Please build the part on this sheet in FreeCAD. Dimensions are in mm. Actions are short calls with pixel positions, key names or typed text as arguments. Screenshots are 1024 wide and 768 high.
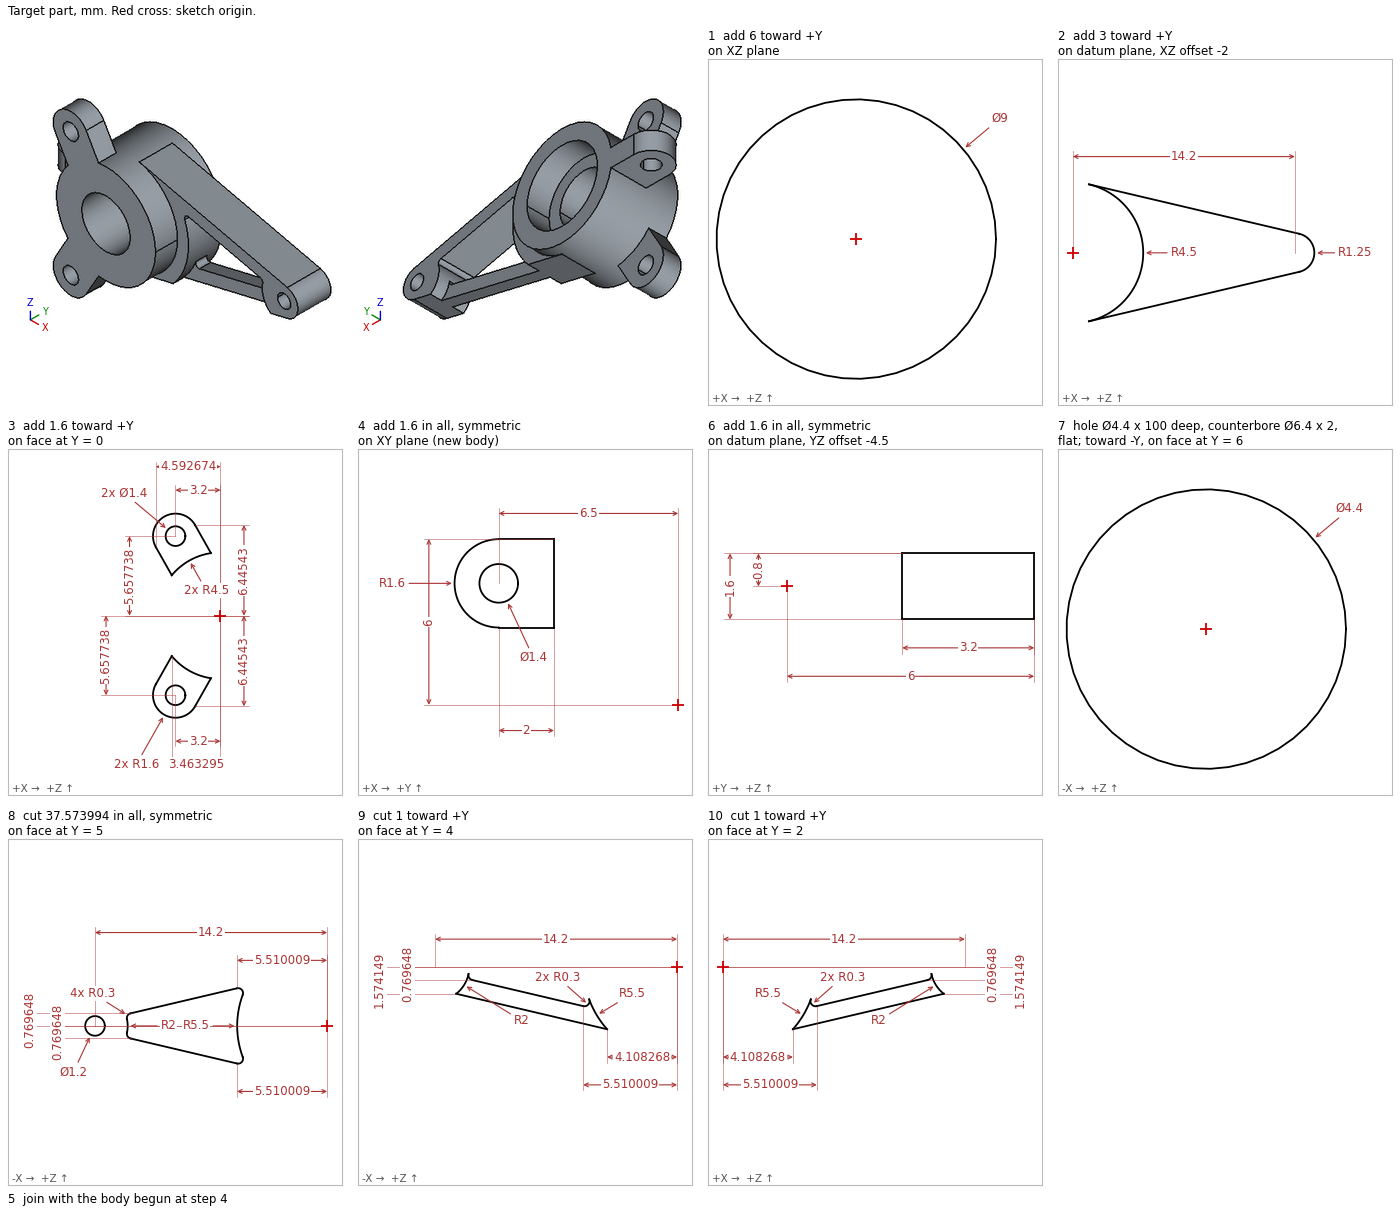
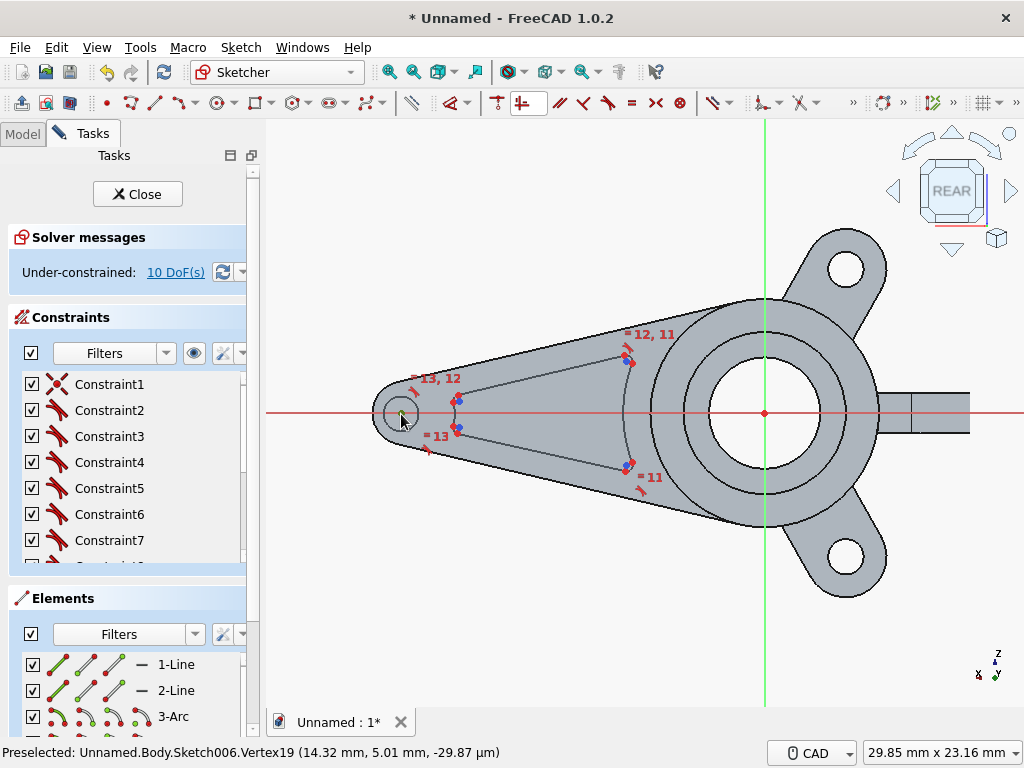
click(334, 413)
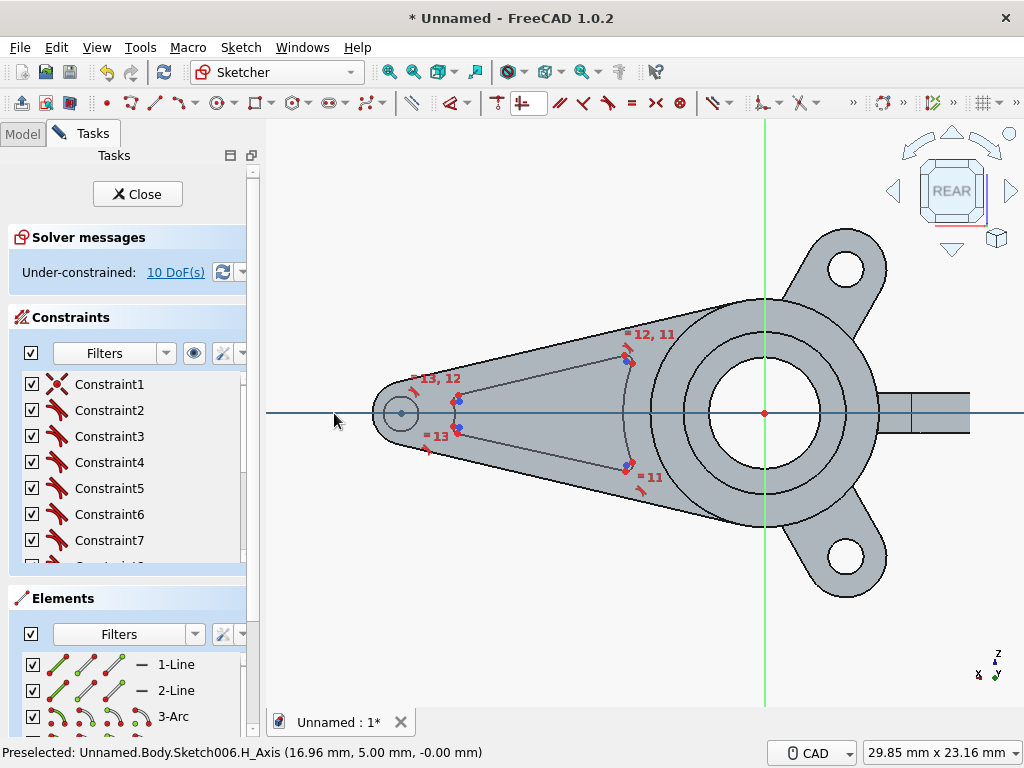
key(c)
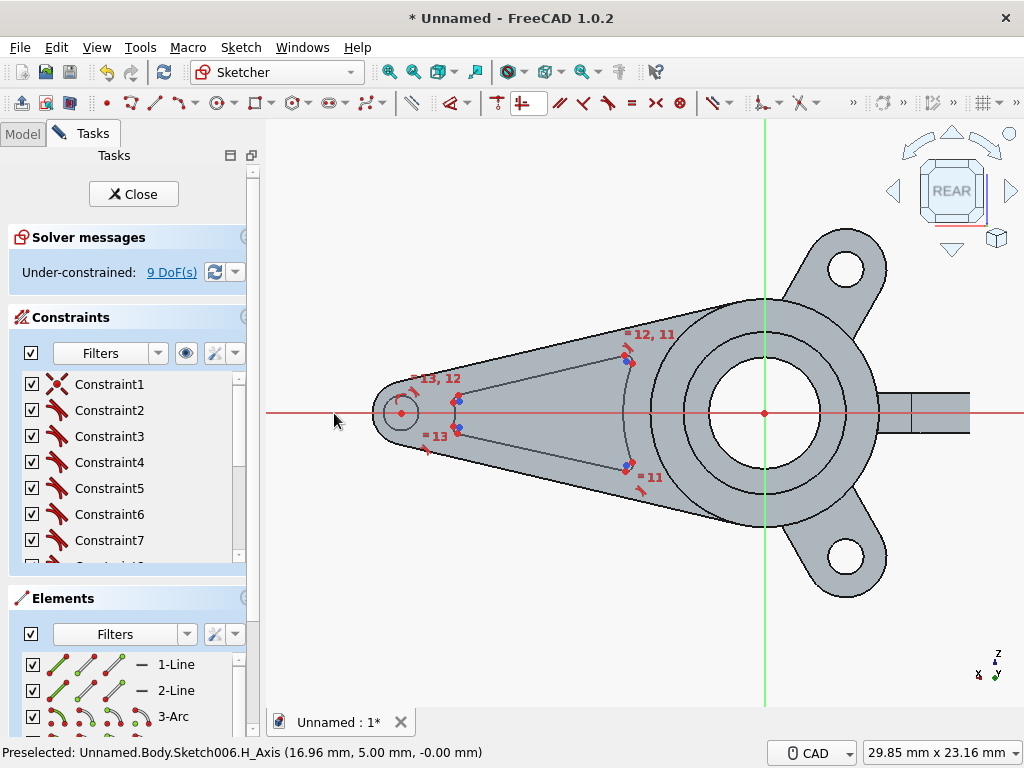
click(450, 104)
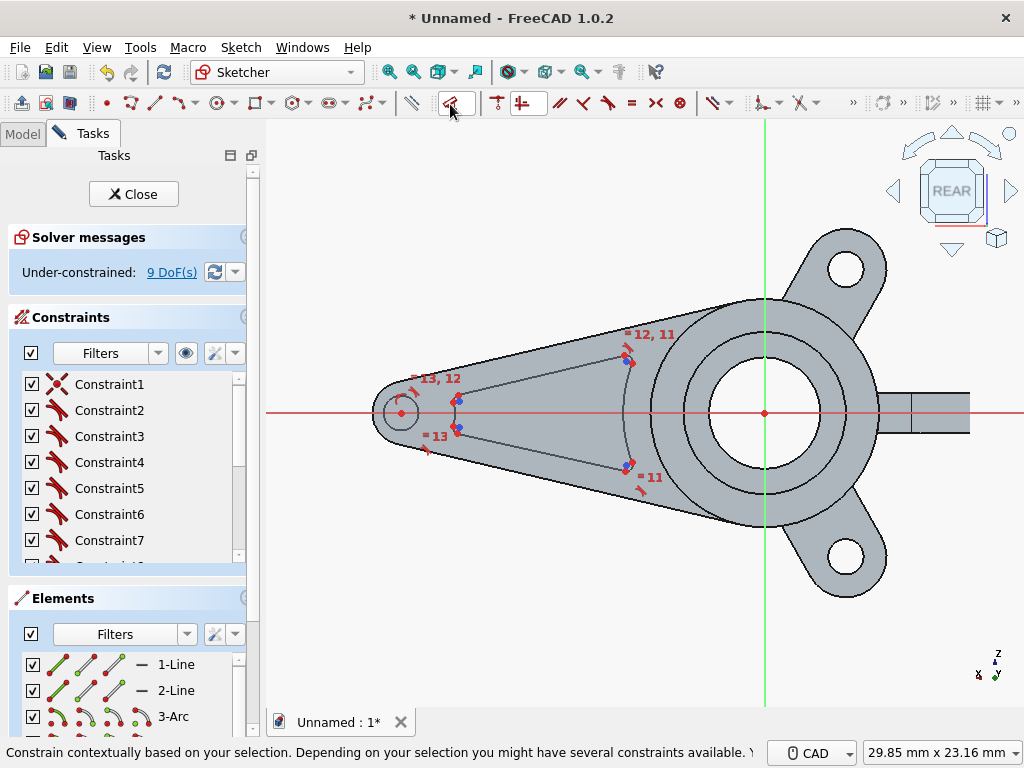
scroll(631, 469, up, 9)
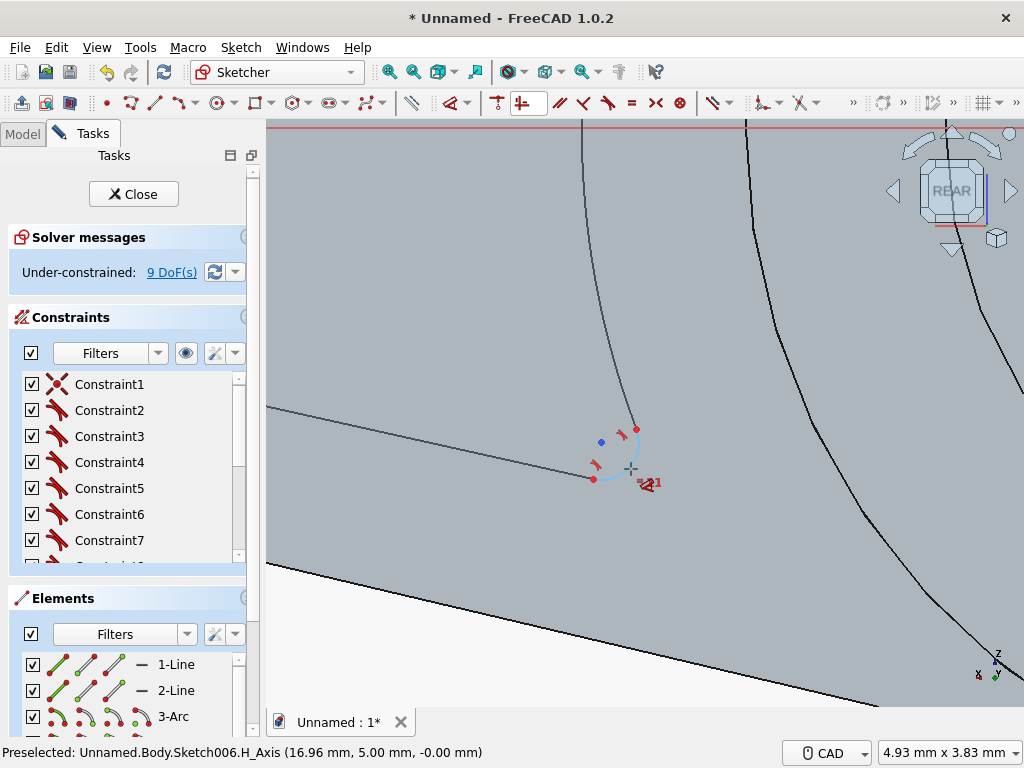
click(630, 467)
click(654, 488)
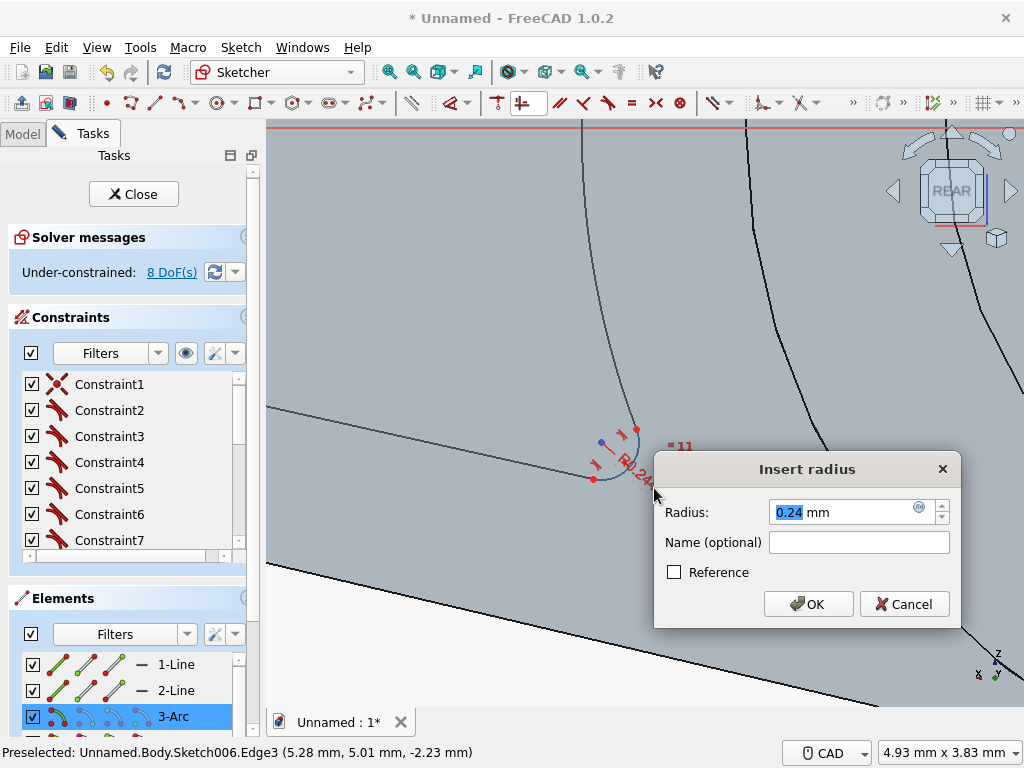
text(0.3)
key(Return)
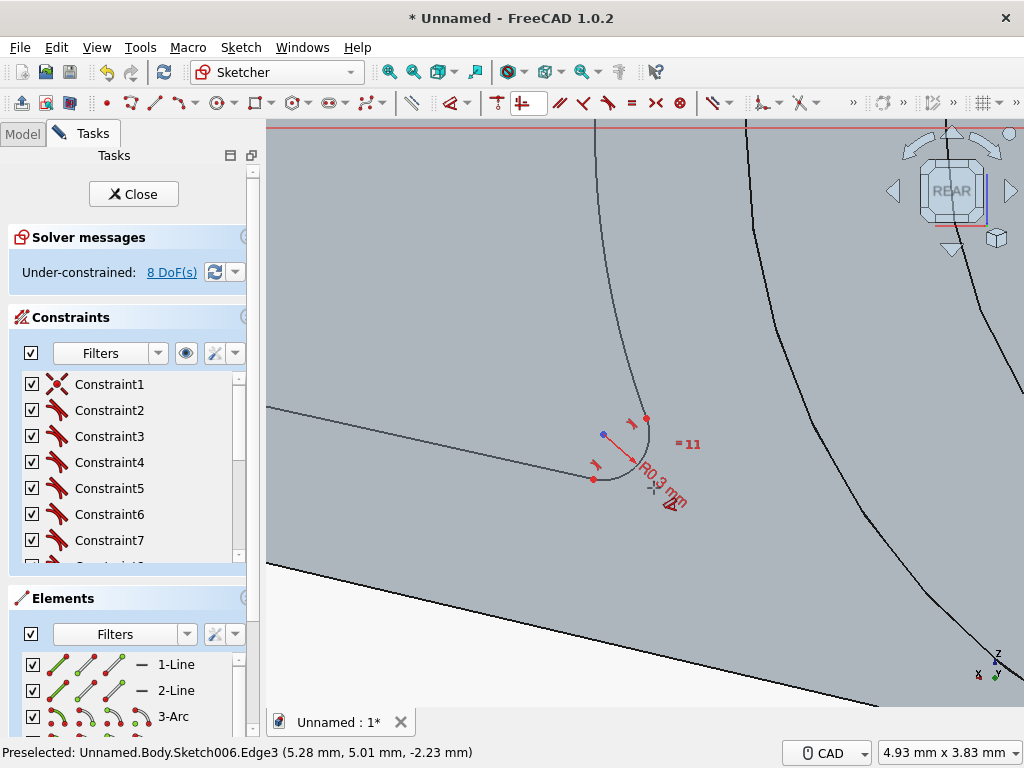
scroll(631, 469, down, 9)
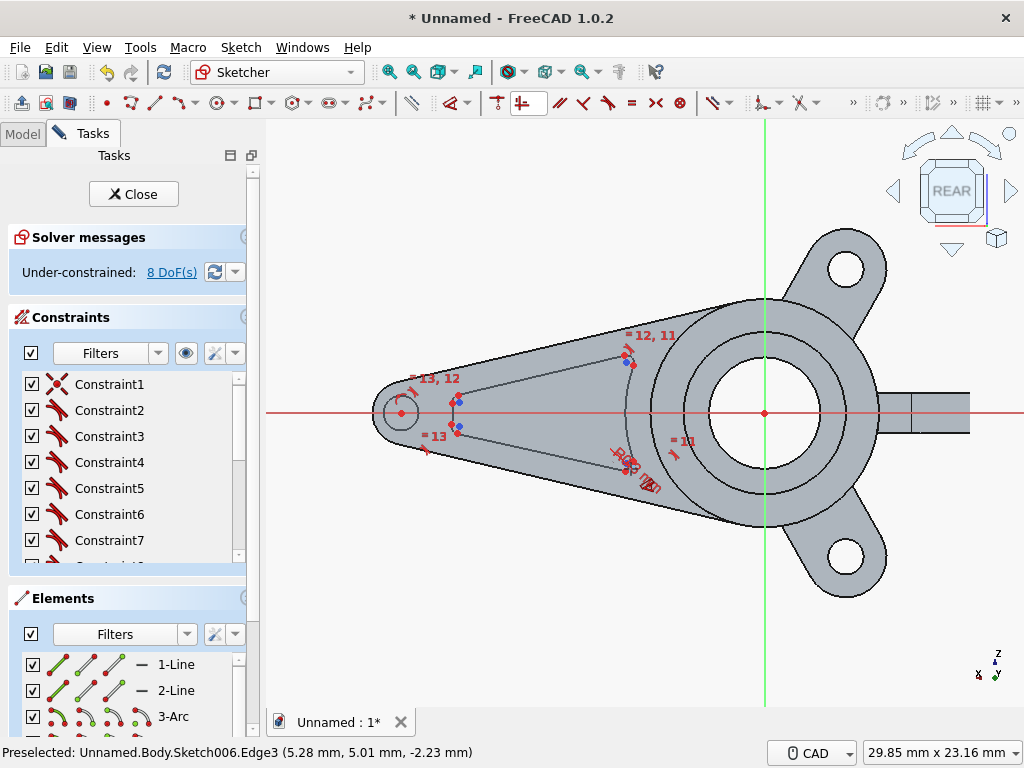
click(627, 433)
click(595, 438)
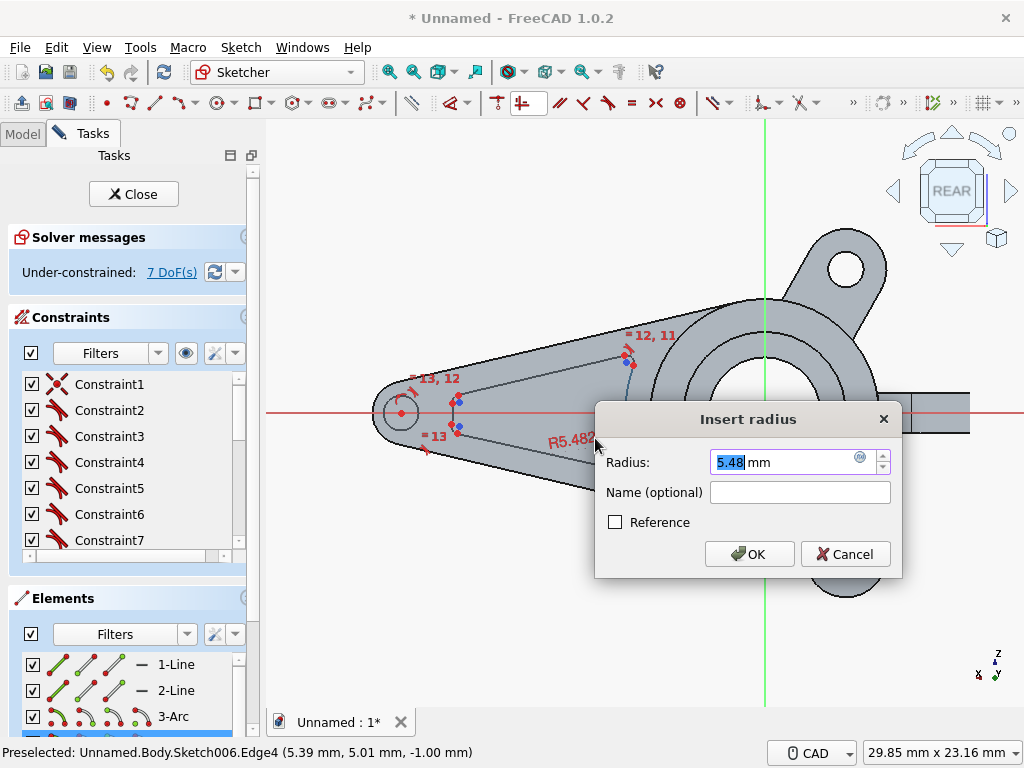
text(5.5)
key(Return)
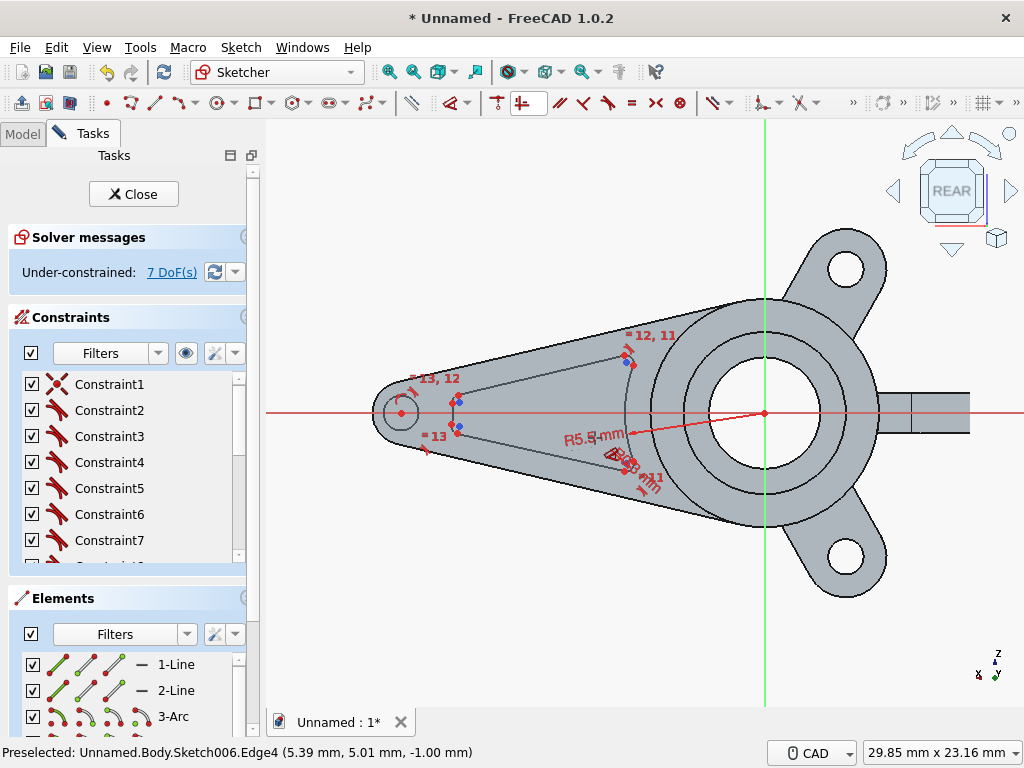
scroll(453, 414, up, 2)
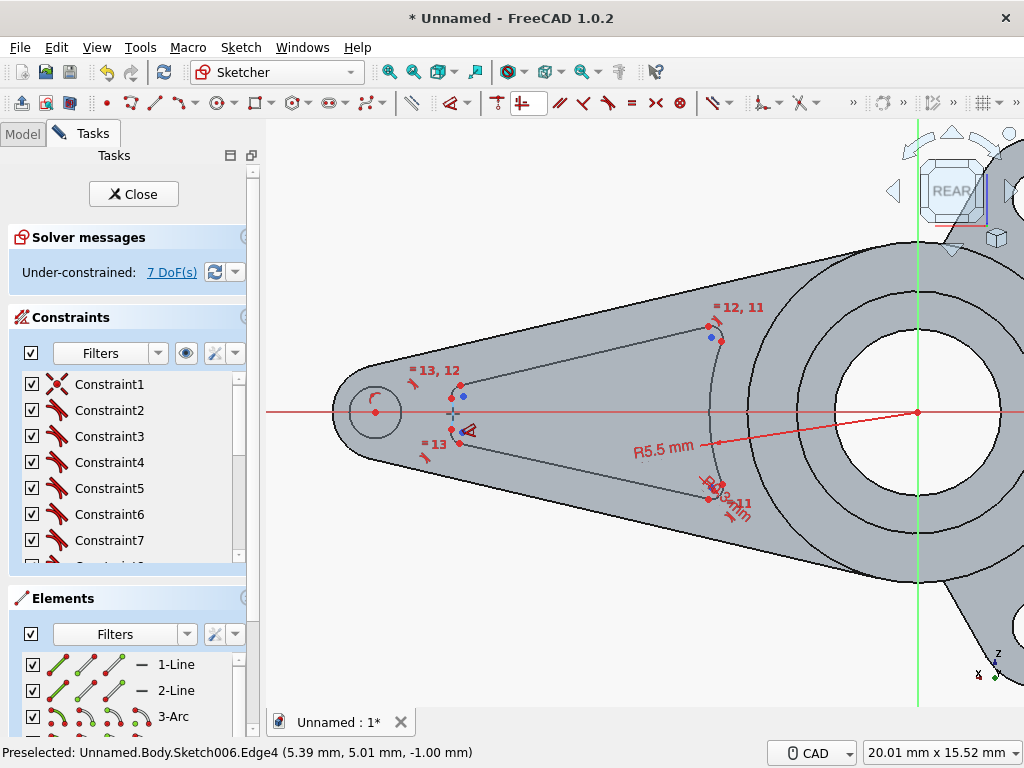
click(453, 414)
click(471, 467)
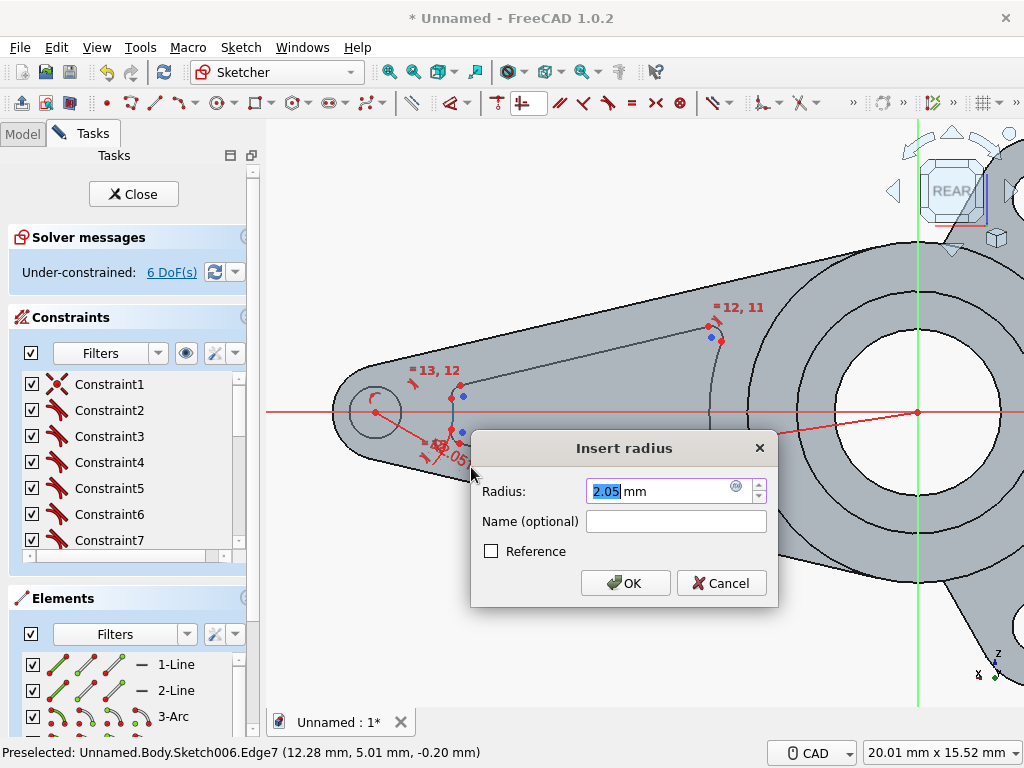
text(2)
key(Return)